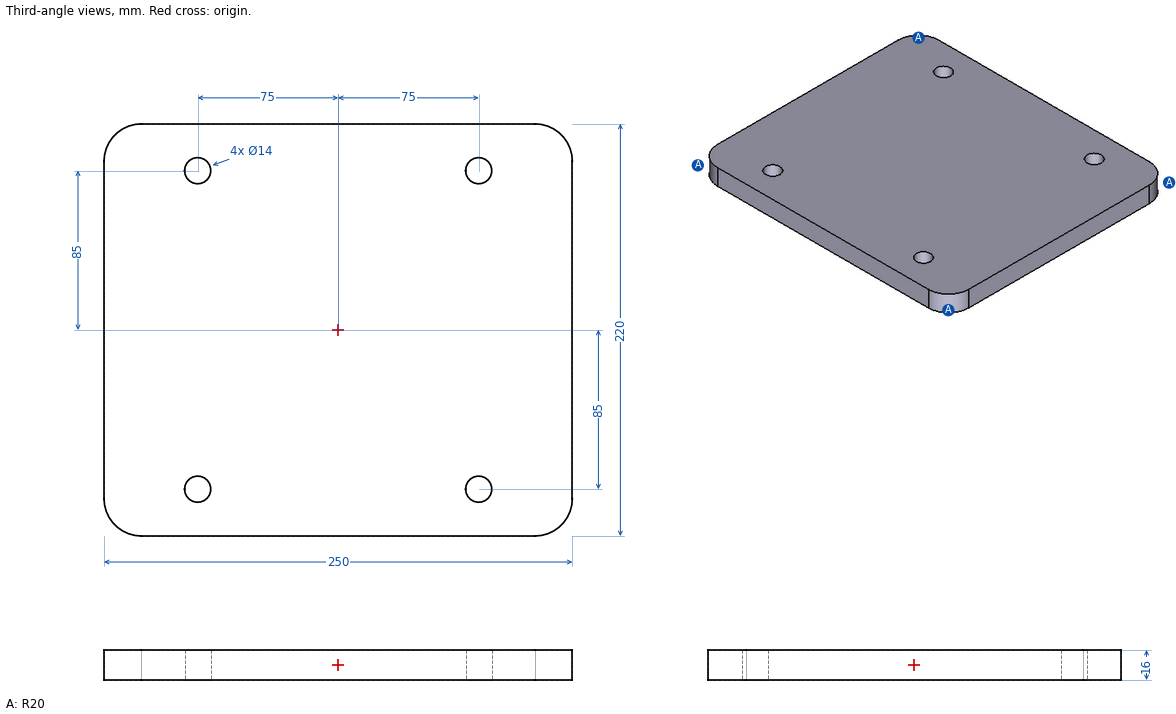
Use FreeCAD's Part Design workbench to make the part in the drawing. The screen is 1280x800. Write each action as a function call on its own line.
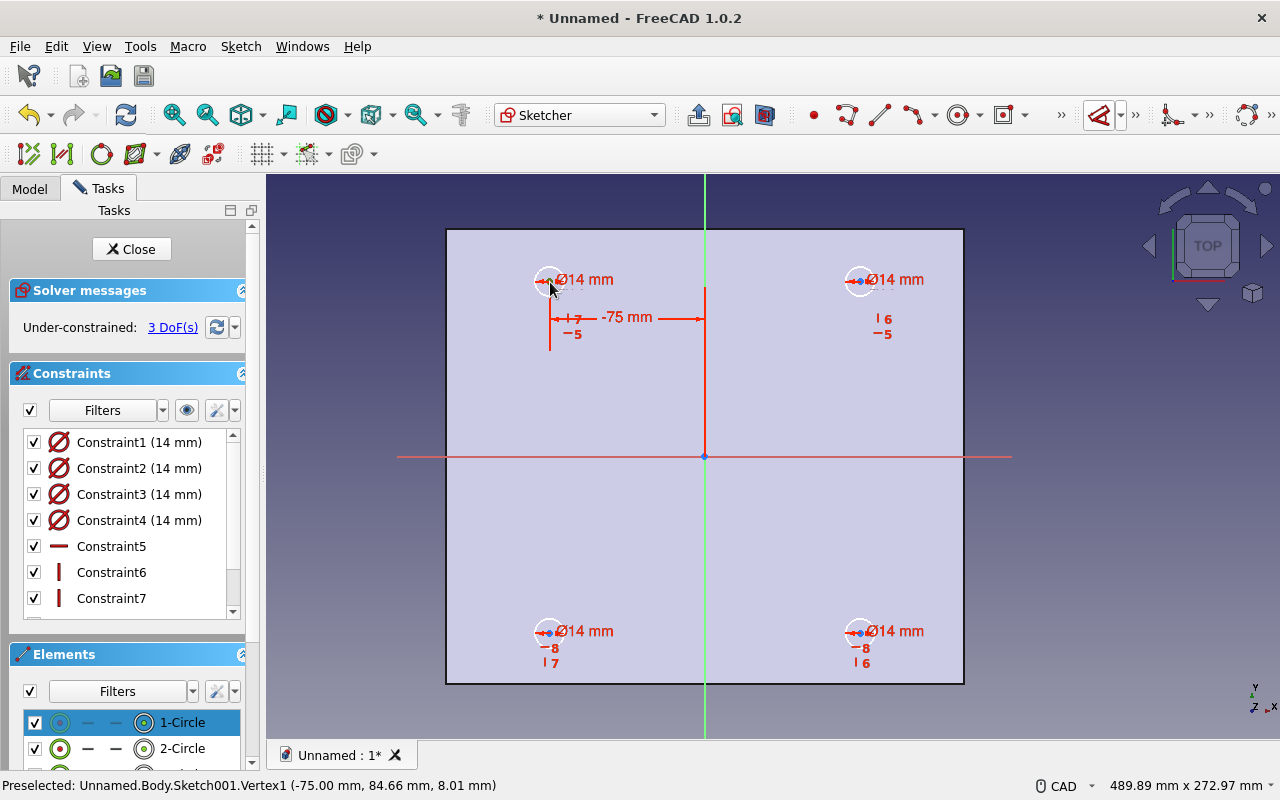
click(1120, 116)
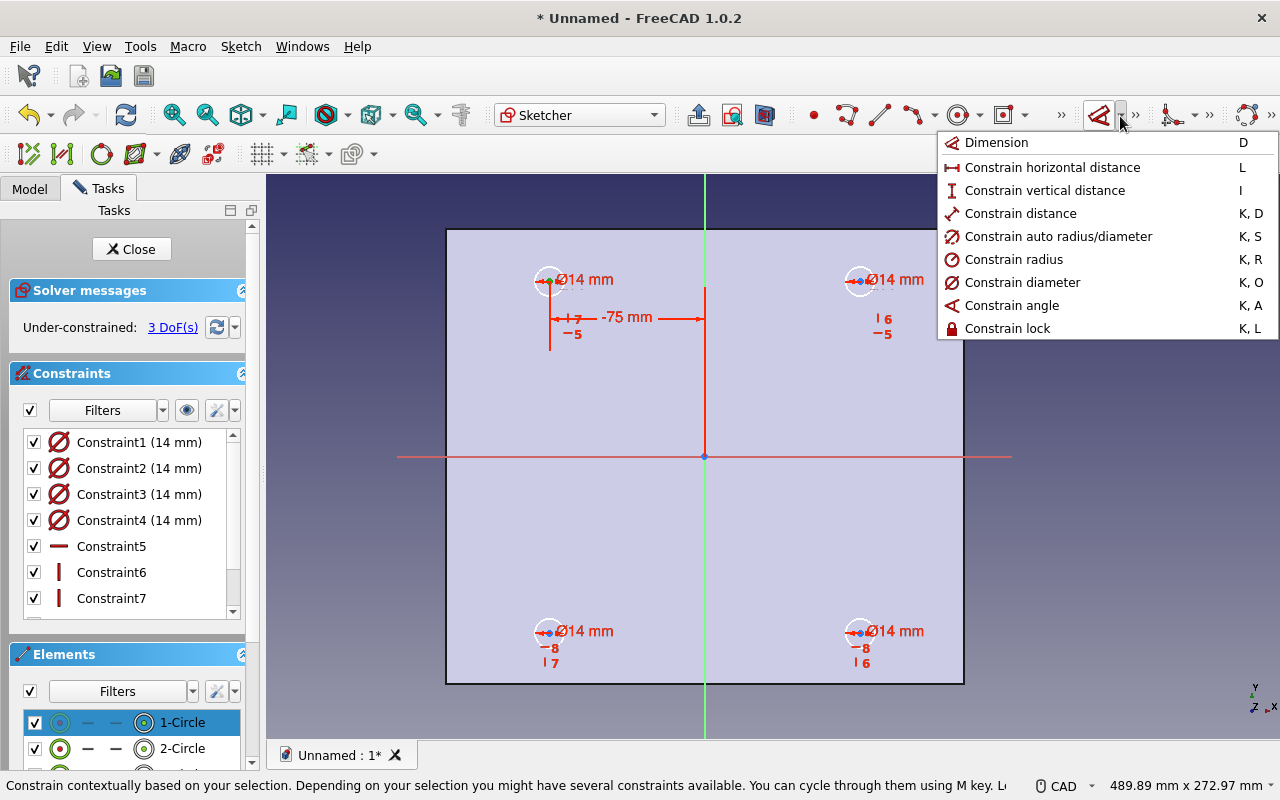
click(1108, 190)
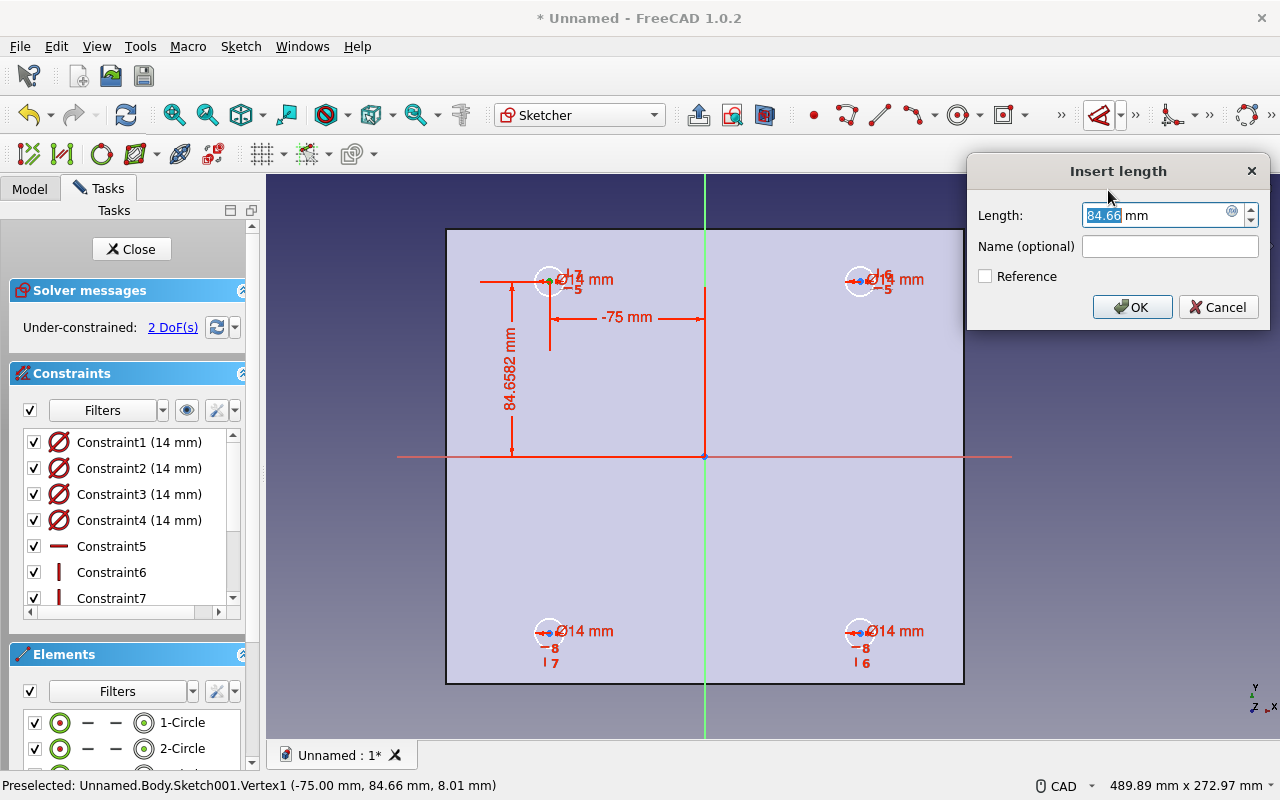
text(85)
key(Return)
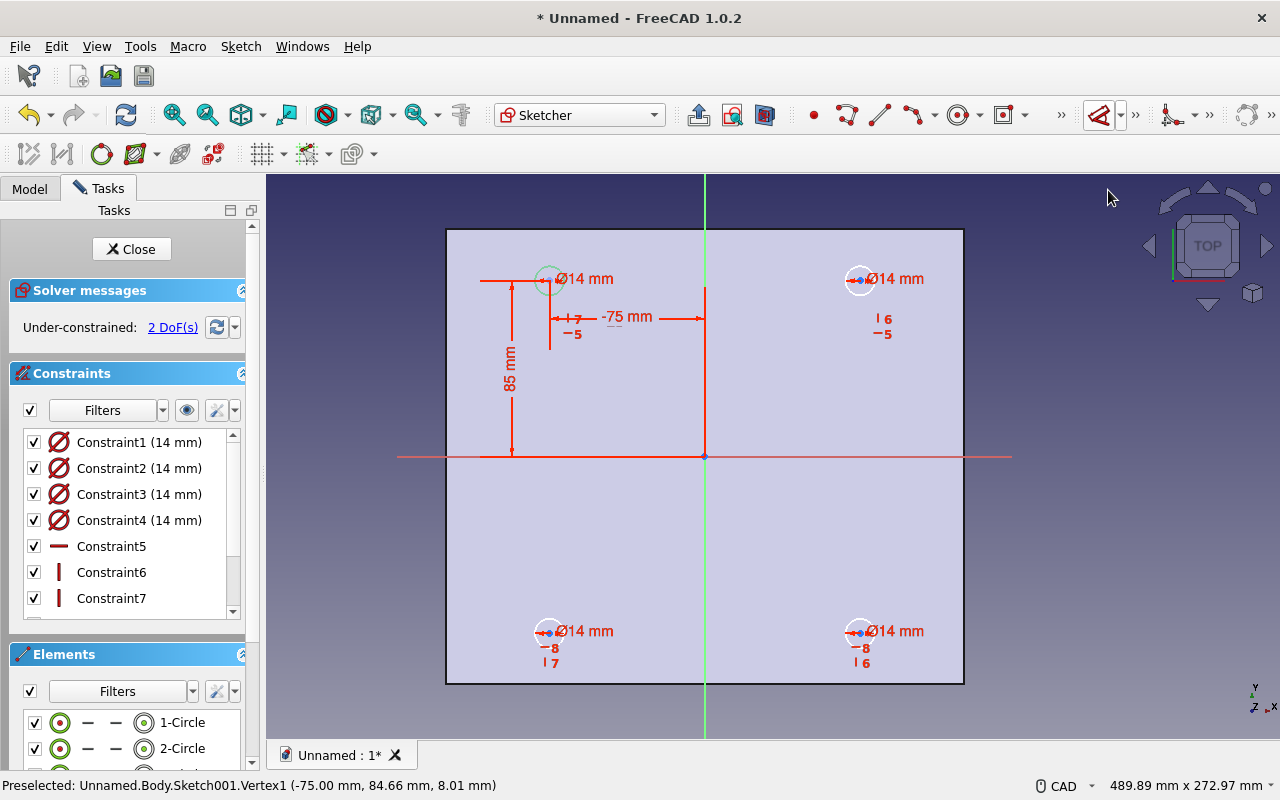
click(860, 281)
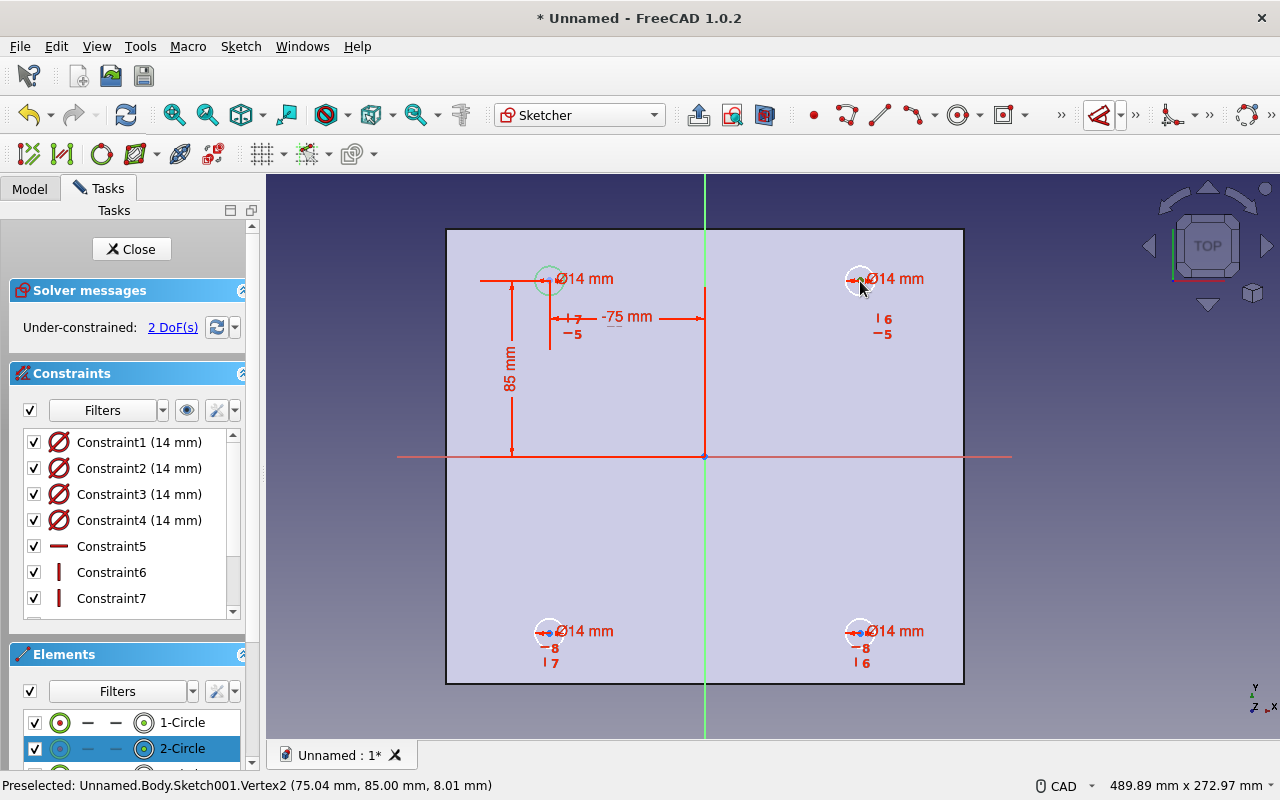
click(1120, 116)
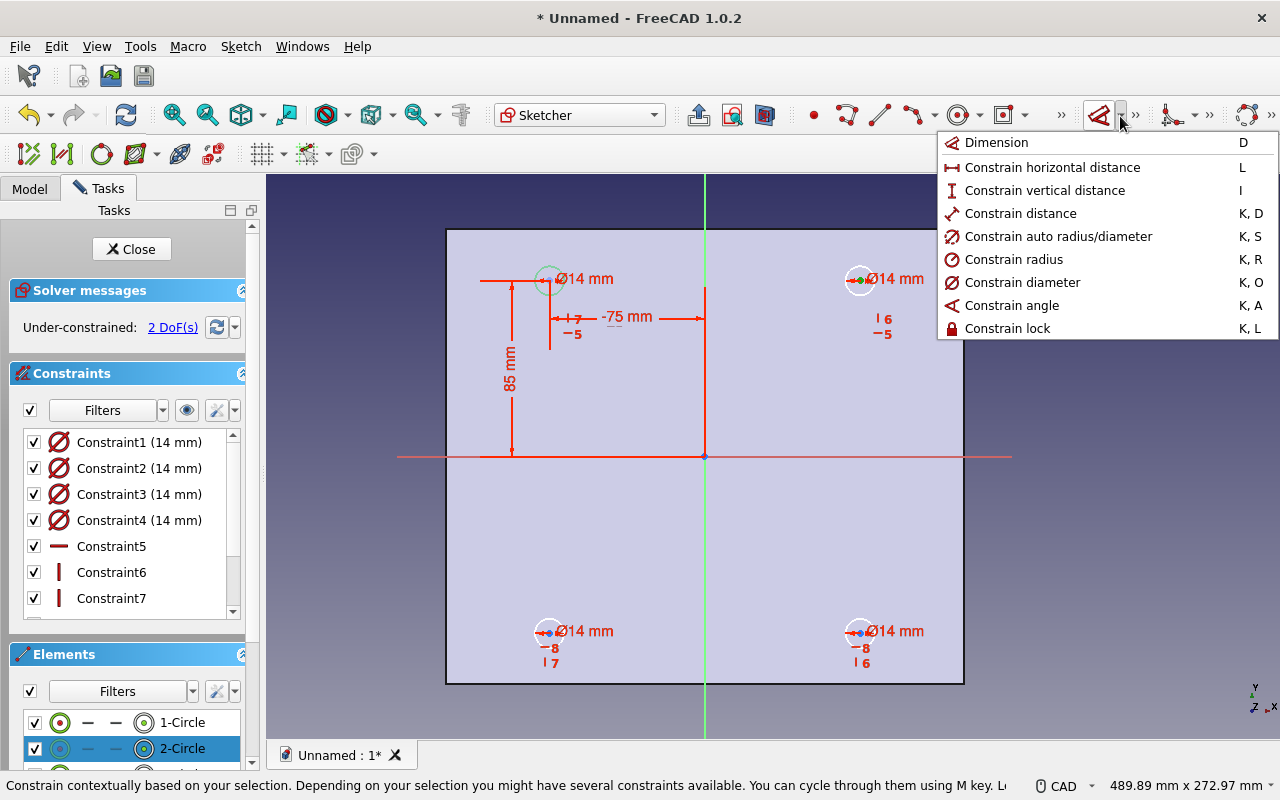
click(1108, 168)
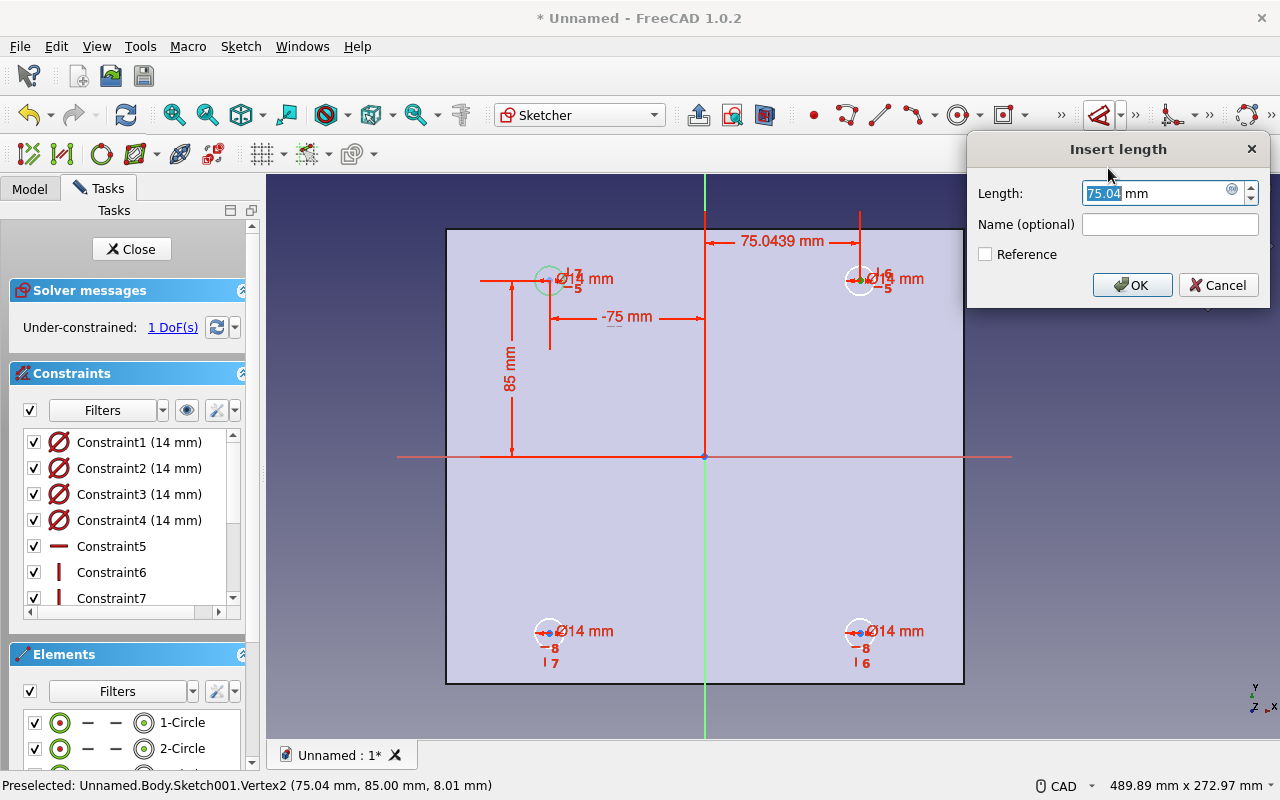
text(75)
key(Return)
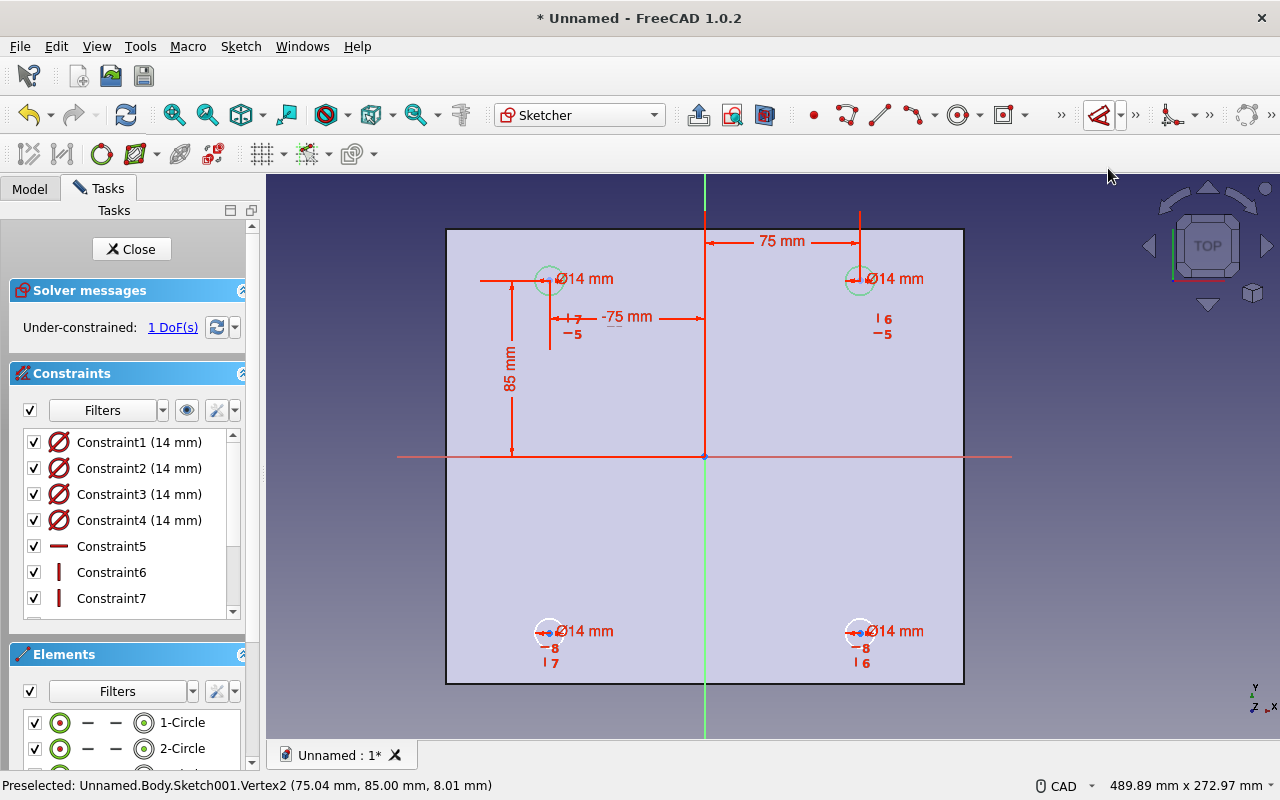
click(860, 633)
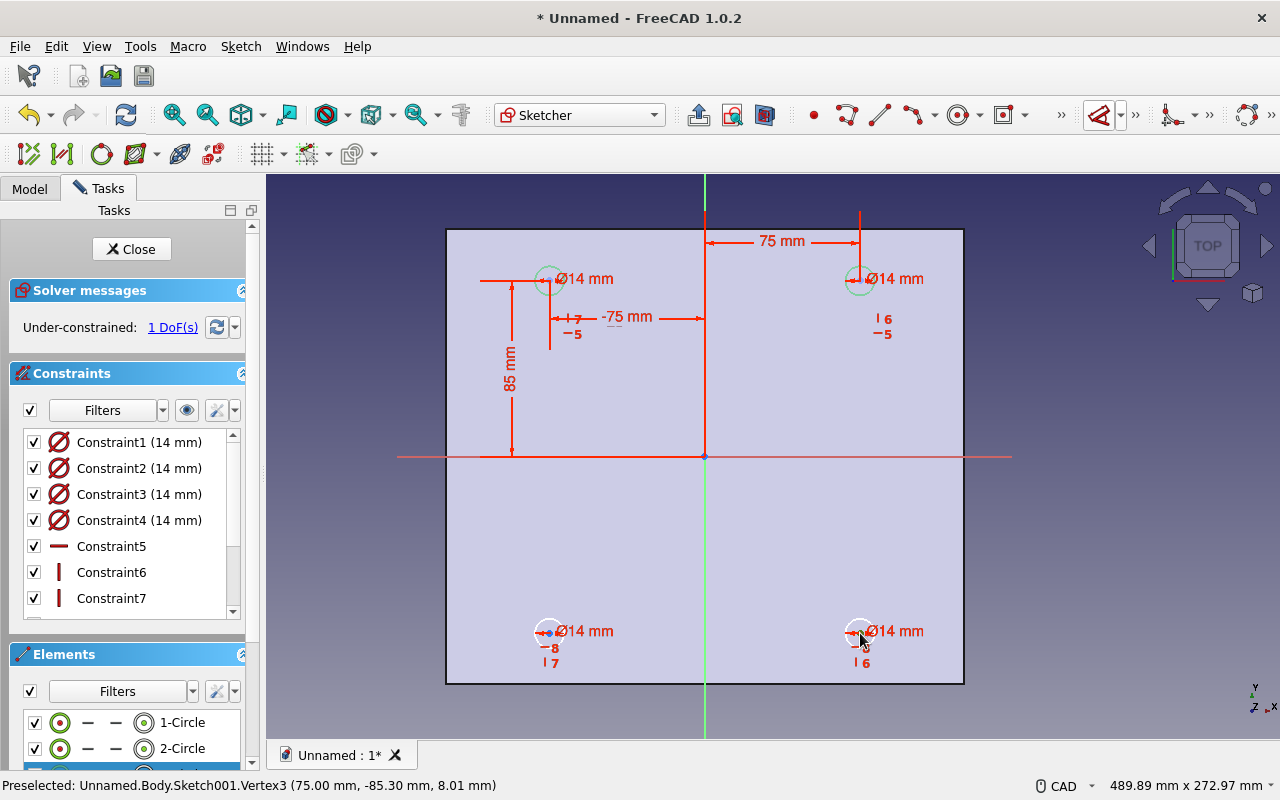
click(1120, 116)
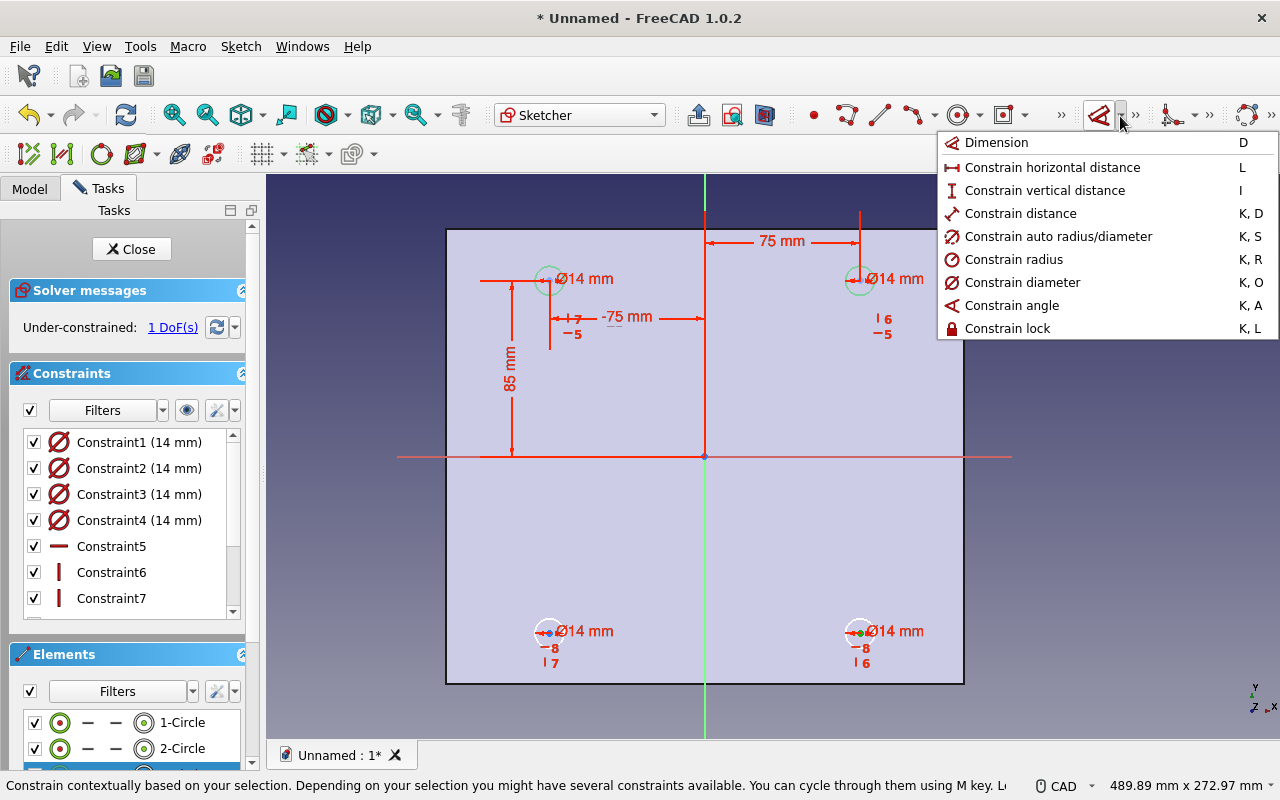
click(1108, 190)